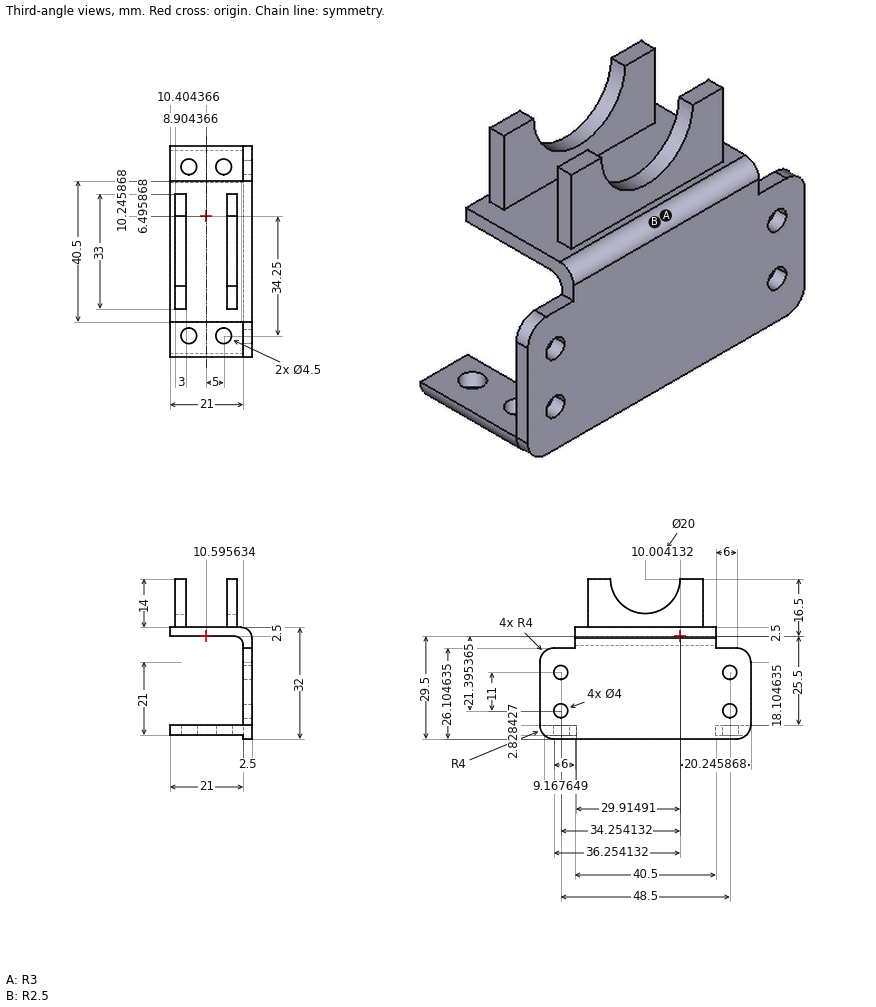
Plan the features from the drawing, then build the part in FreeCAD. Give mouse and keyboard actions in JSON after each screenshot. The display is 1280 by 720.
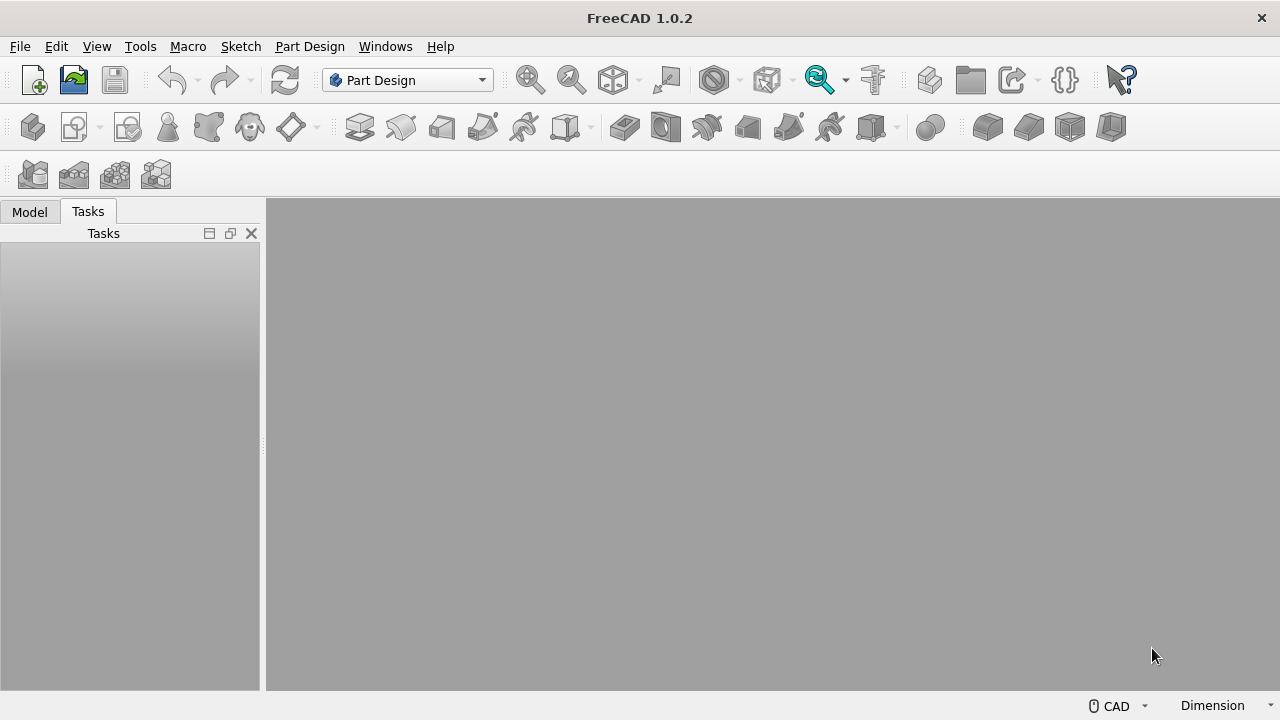
{"action": "left_click", "coordinate": [33, 80]}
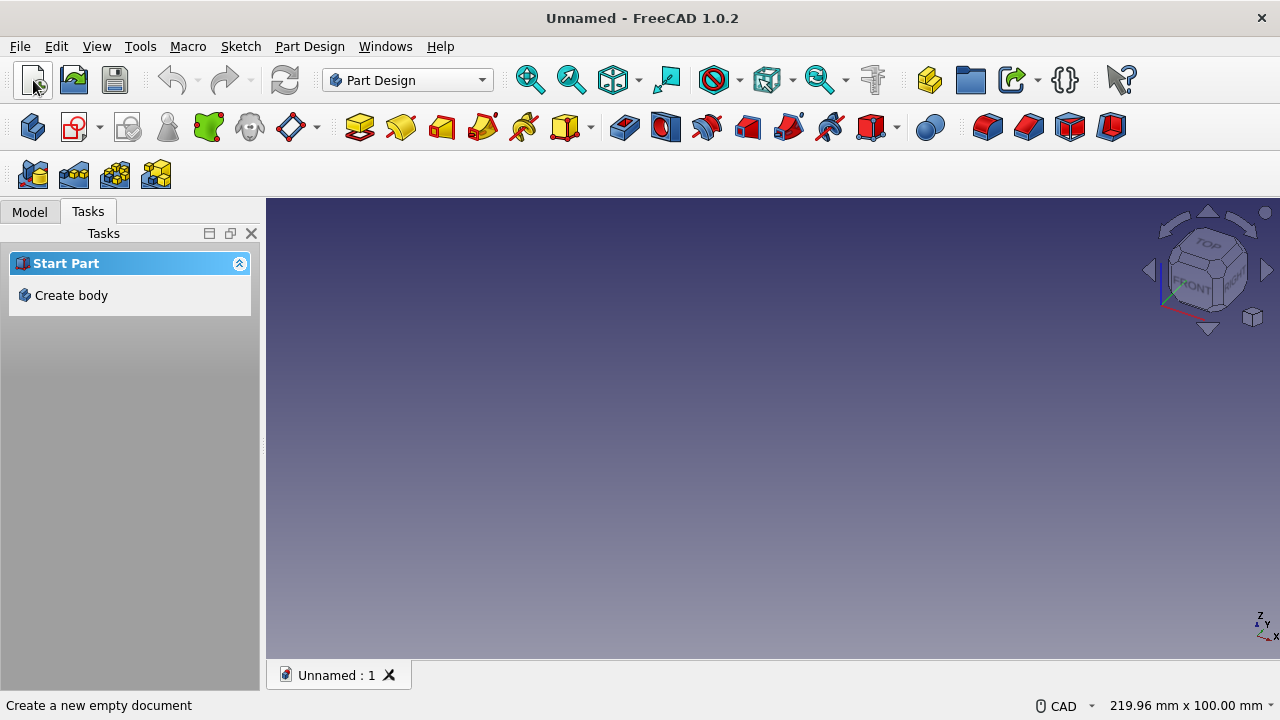
{"action": "left_click", "coordinate": [74, 128]}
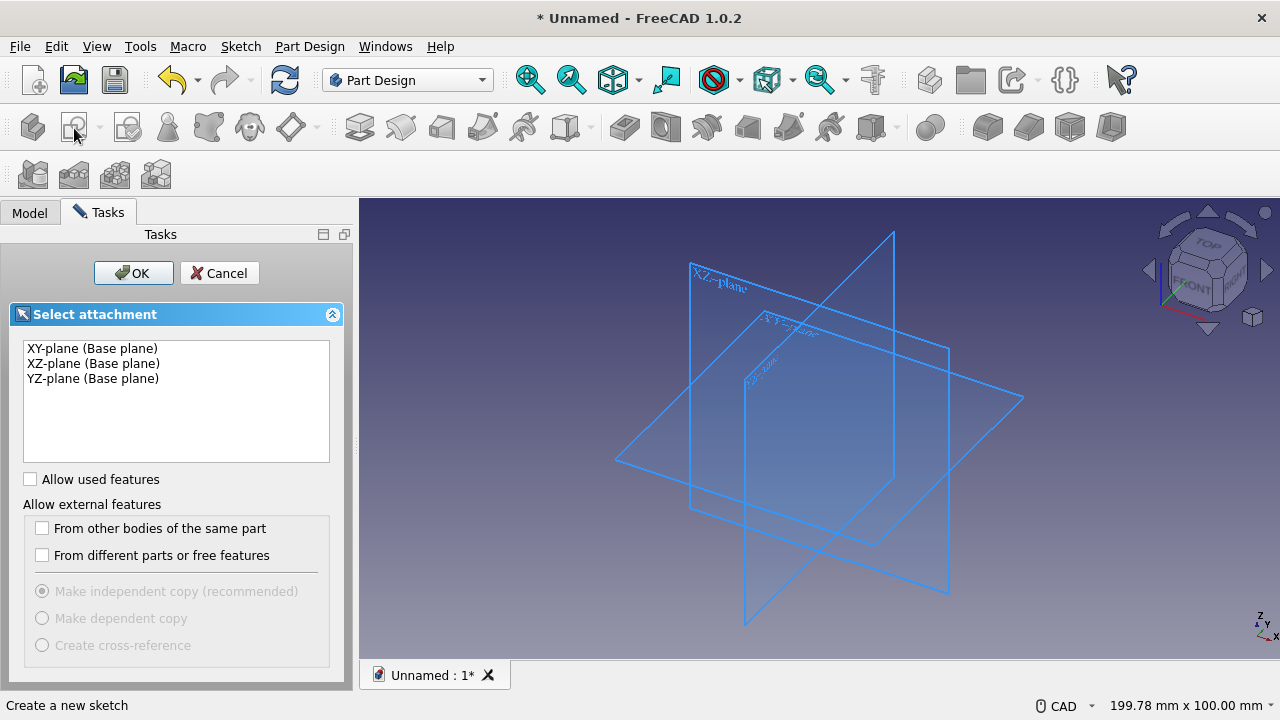
{"action": "left_click", "coordinate": [84, 348]}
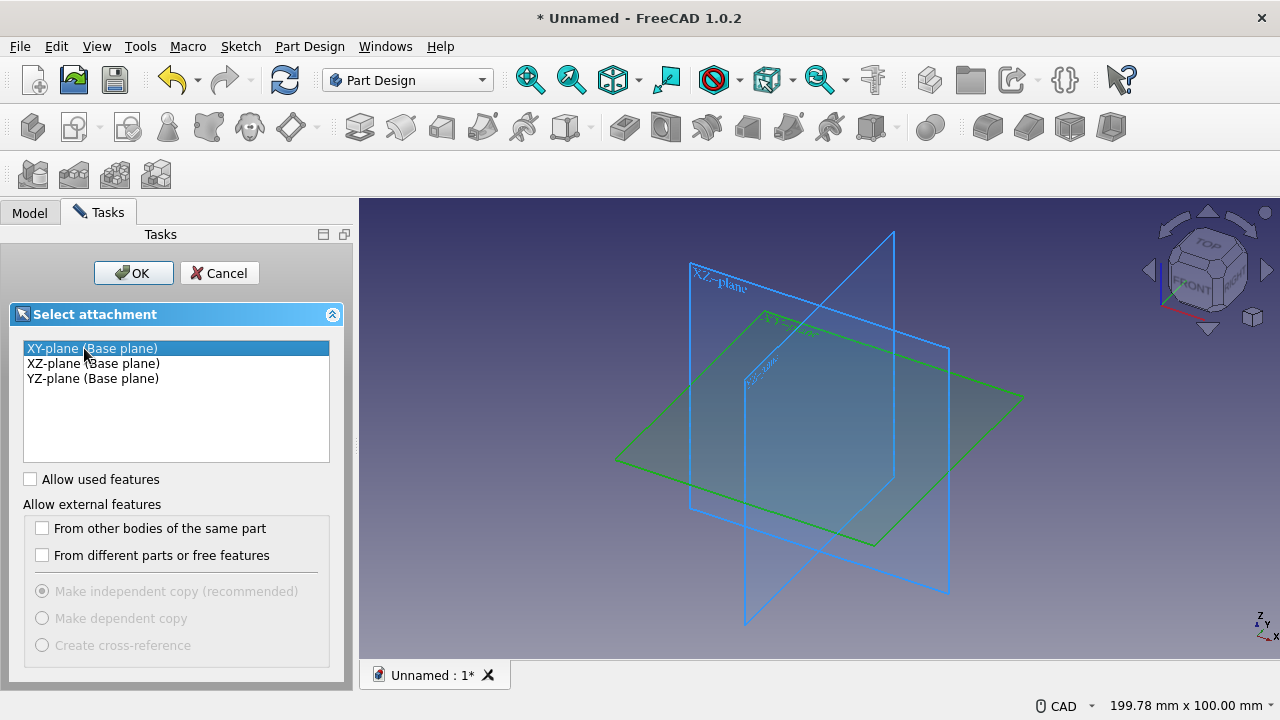
{"action": "left_click", "coordinate": [134, 273]}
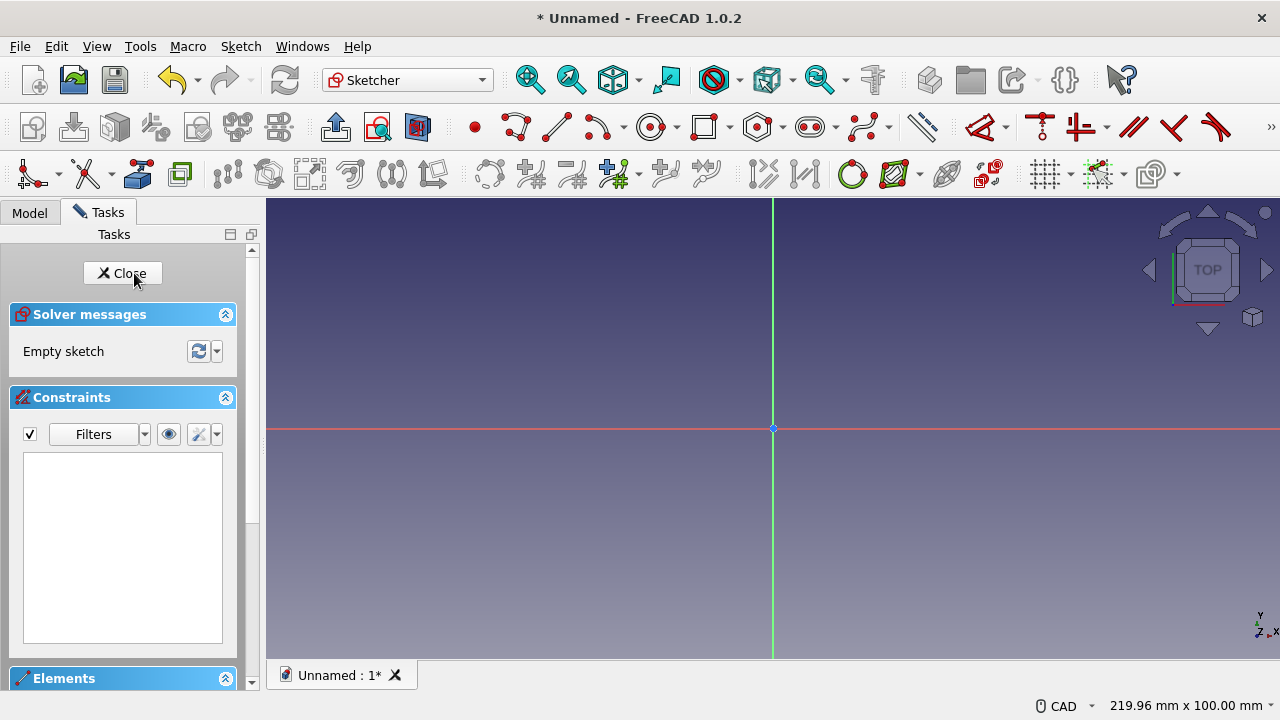
{"action": "scroll", "coordinate": [914, 568], "scroll_direction": "up", "scroll_amount": 2}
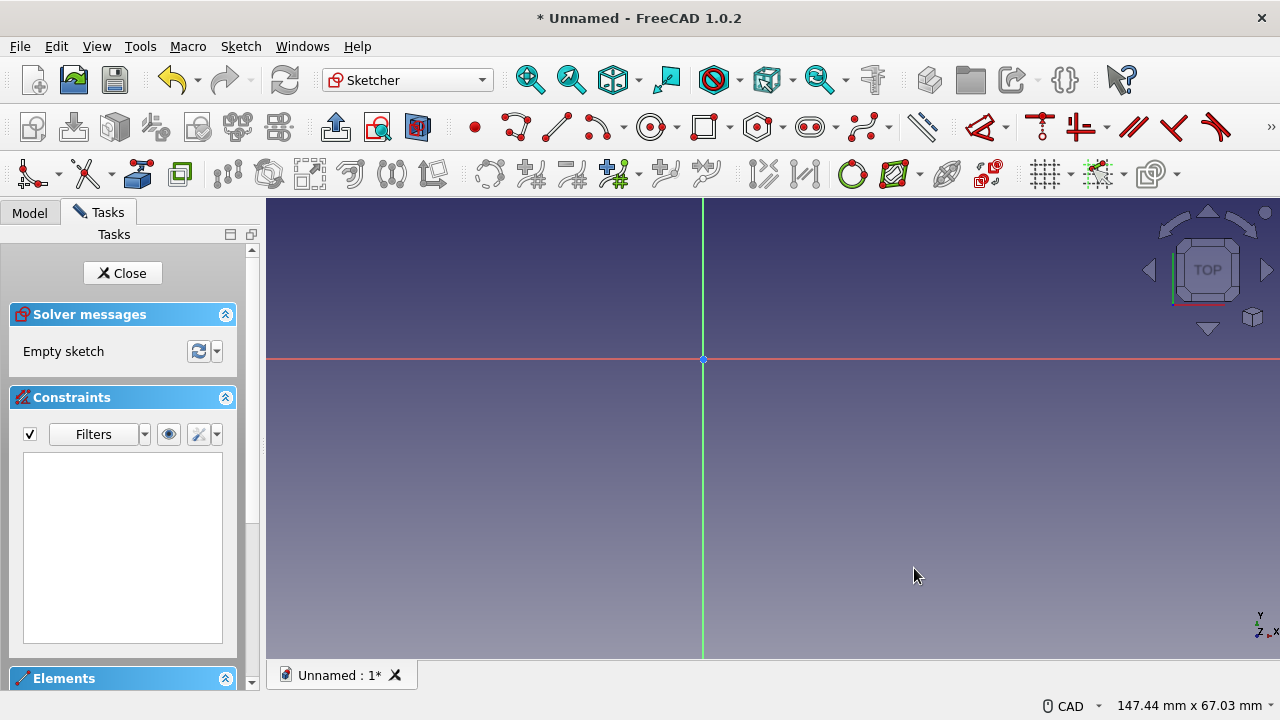
{"action": "left_click", "coordinate": [704, 128]}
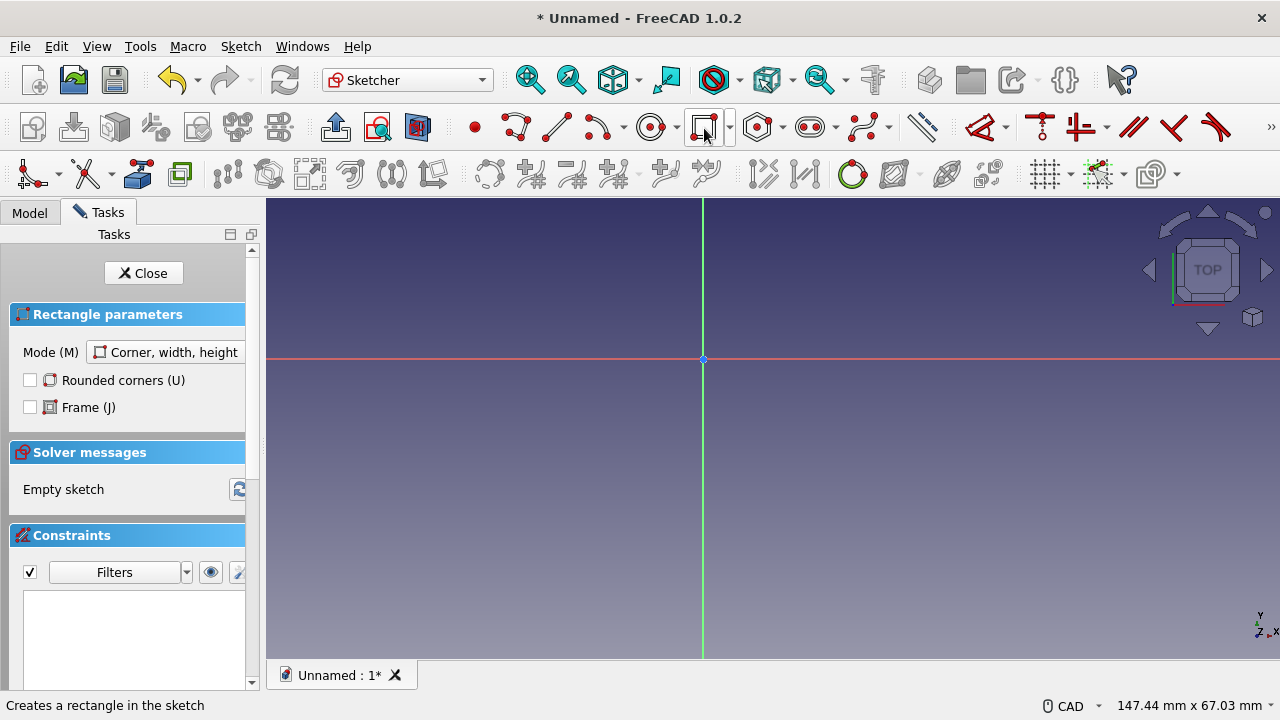
{"action": "left_click", "coordinate": [632, 289]}
{"action": "left_click", "coordinate": [776, 568]}
{"action": "key", "text": "Escape"}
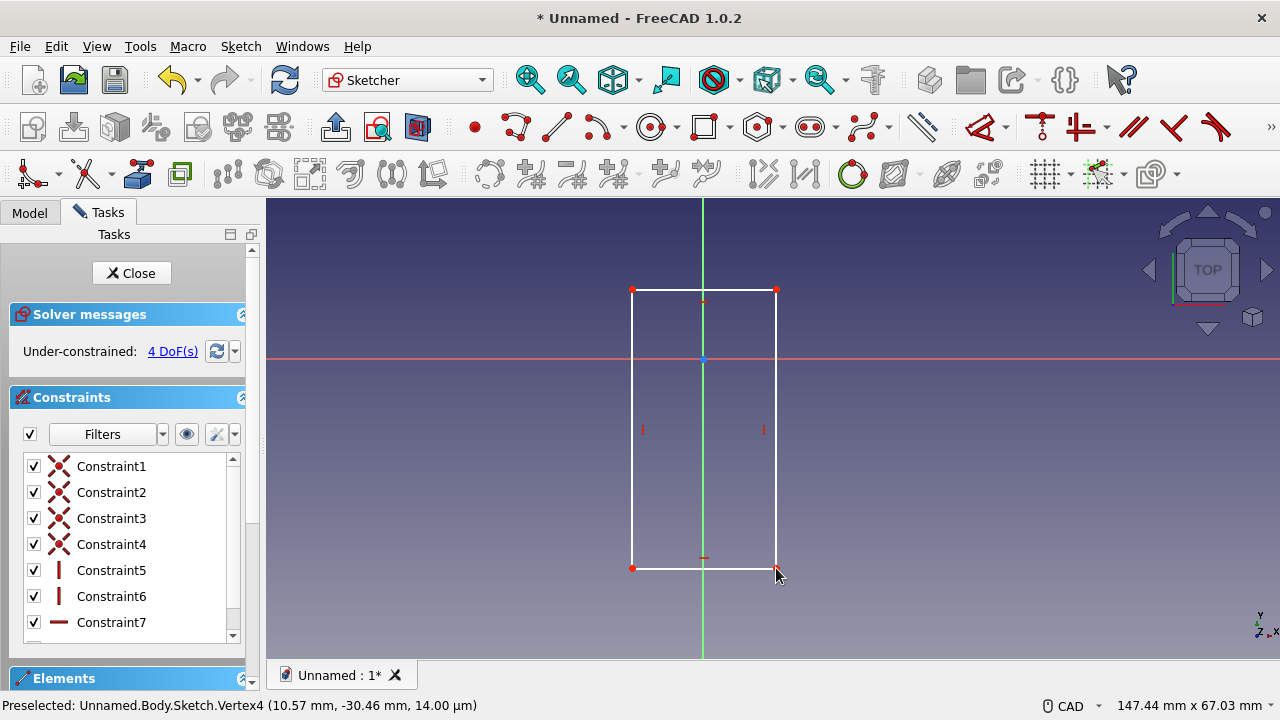
{"action": "left_click", "coordinate": [980, 128]}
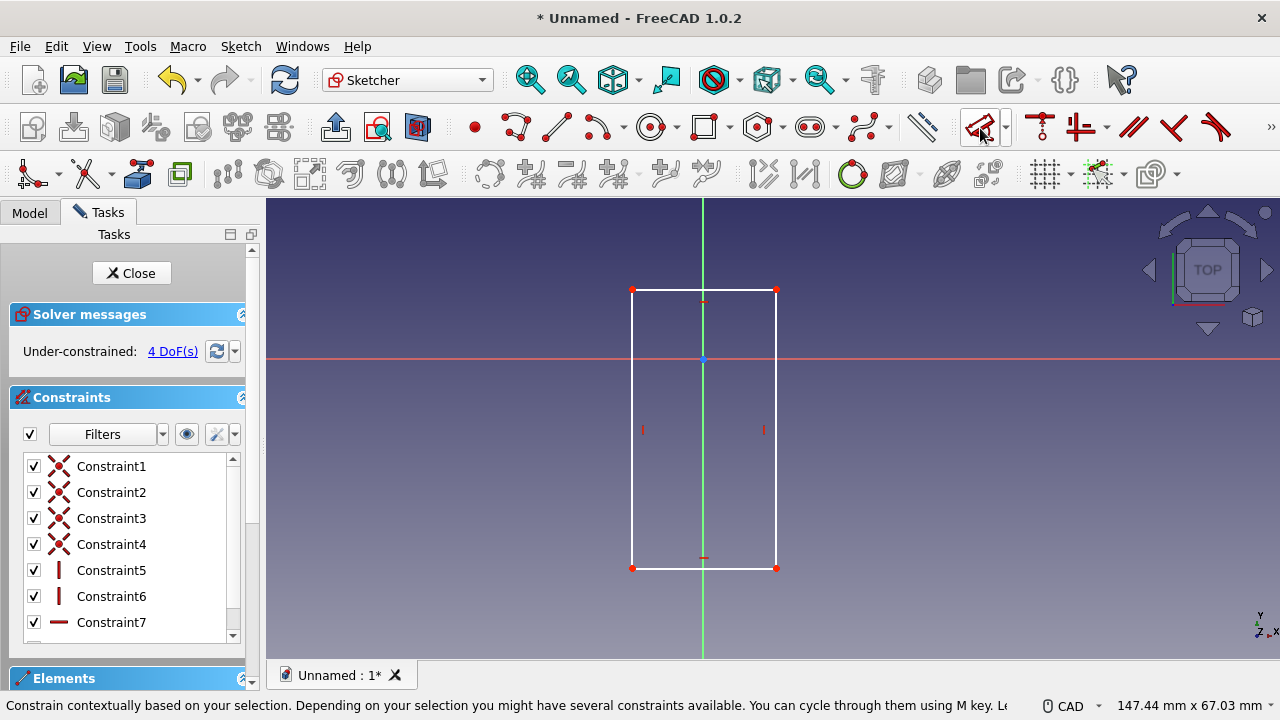
{"action": "left_click", "coordinate": [675, 569]}
{"action": "left_click", "coordinate": [671, 603]}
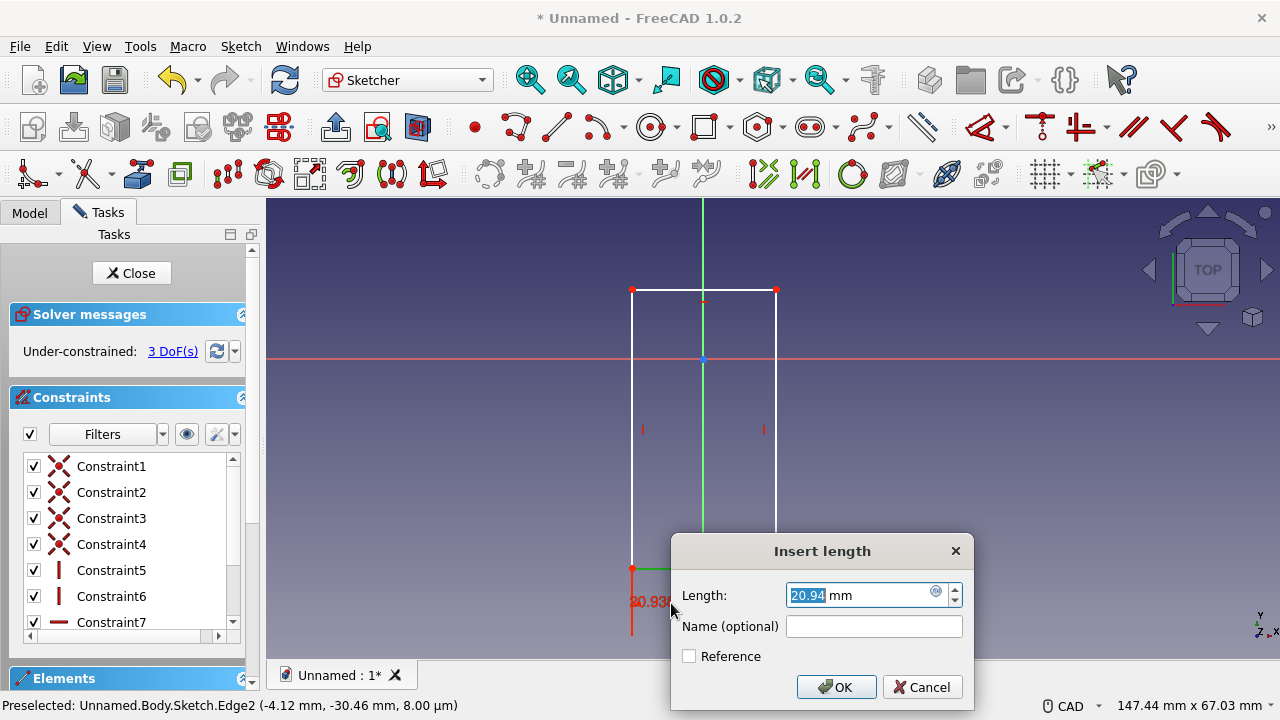
{"action": "type", "text": "21"}
{"action": "key", "text": "Return"}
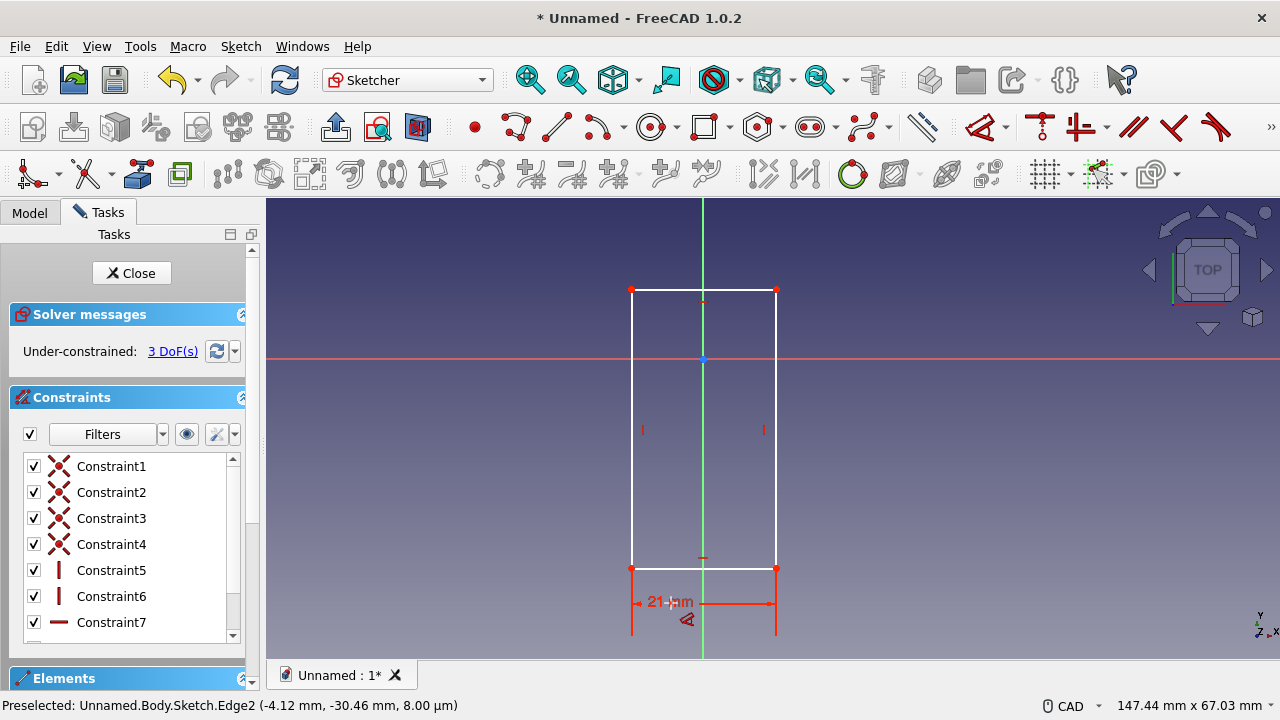
{"action": "left_click", "coordinate": [632, 374]}
{"action": "left_click", "coordinate": [598, 429]}